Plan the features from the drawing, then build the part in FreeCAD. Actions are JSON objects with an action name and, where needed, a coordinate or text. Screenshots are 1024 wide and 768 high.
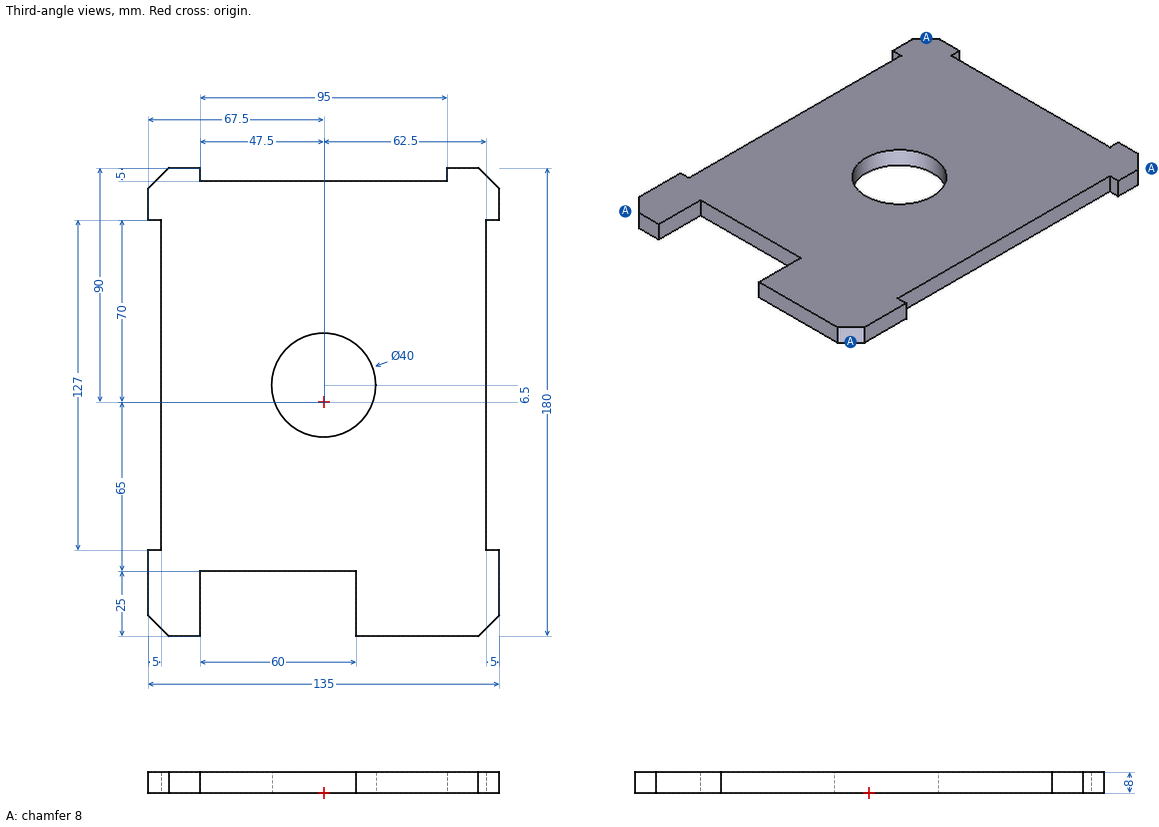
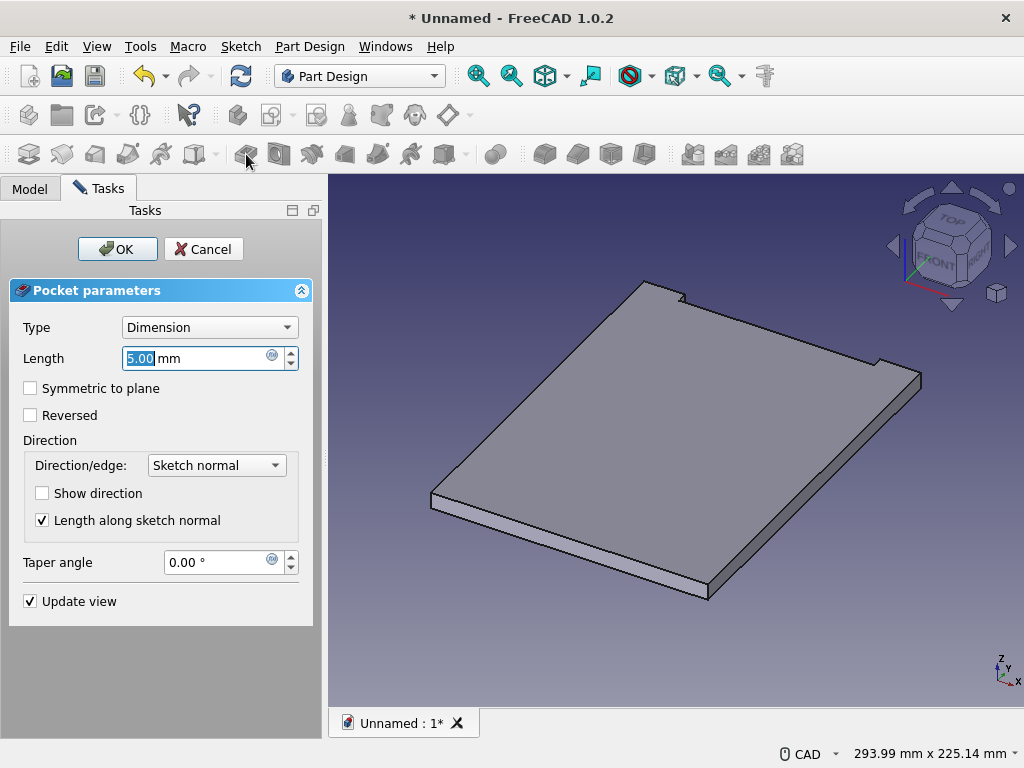
{"action": "left_click", "coordinate": [210, 328]}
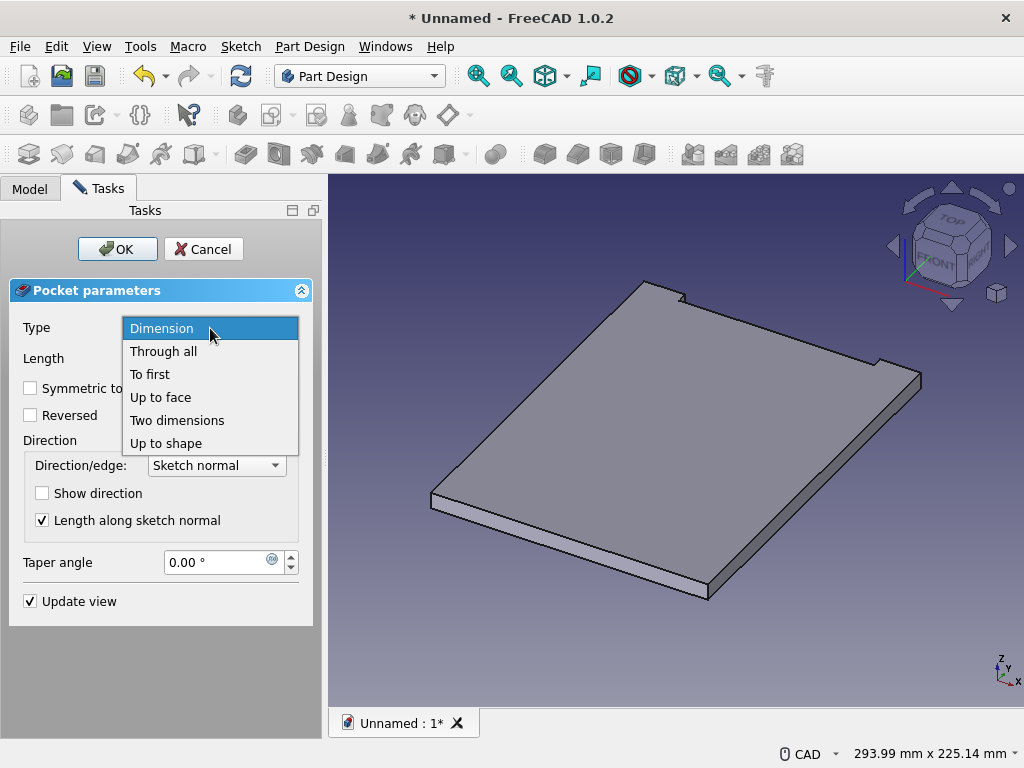
{"action": "left_click", "coordinate": [208, 374]}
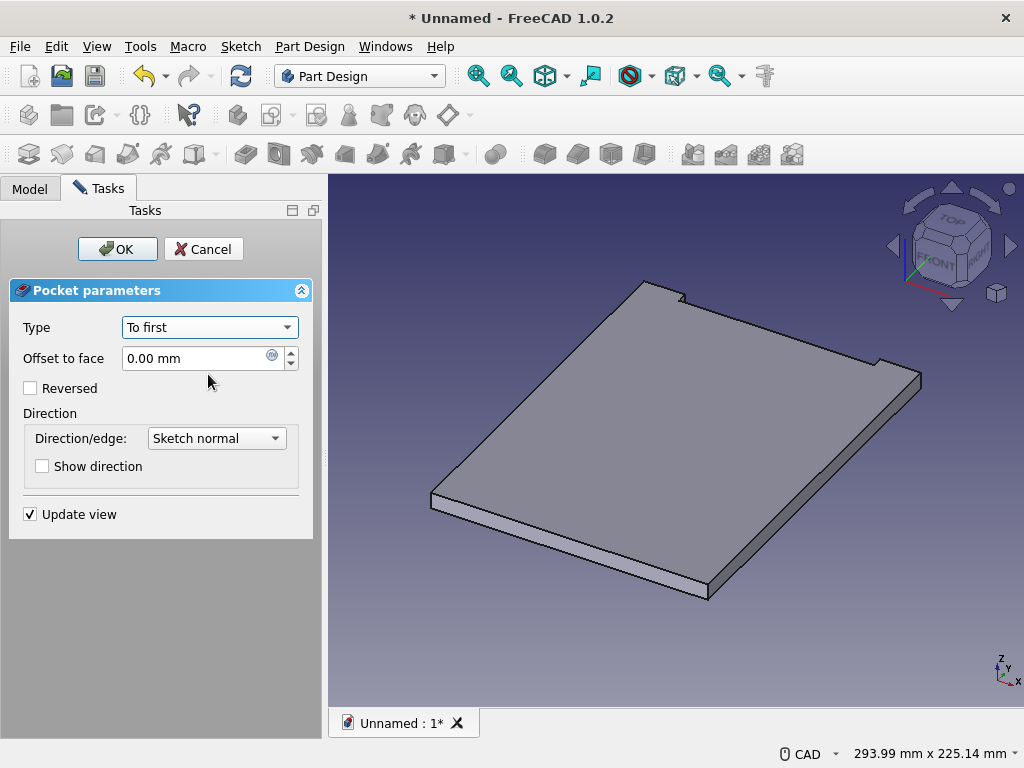
{"action": "left_click", "coordinate": [118, 249]}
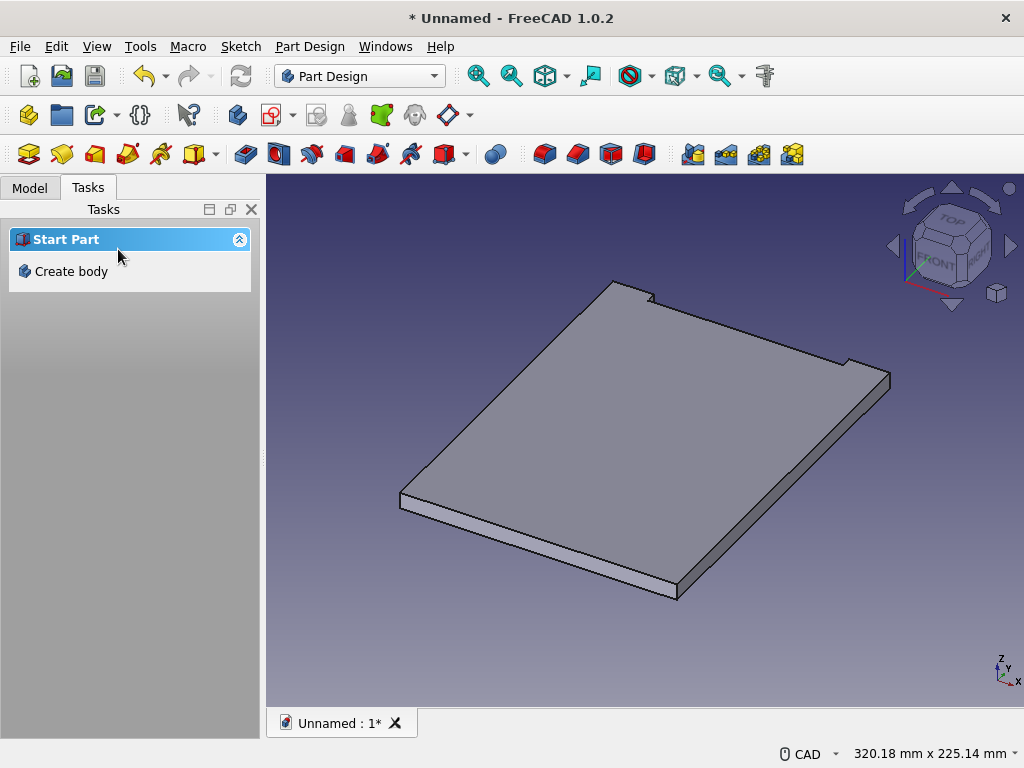
{"action": "left_click", "coordinate": [645, 432]}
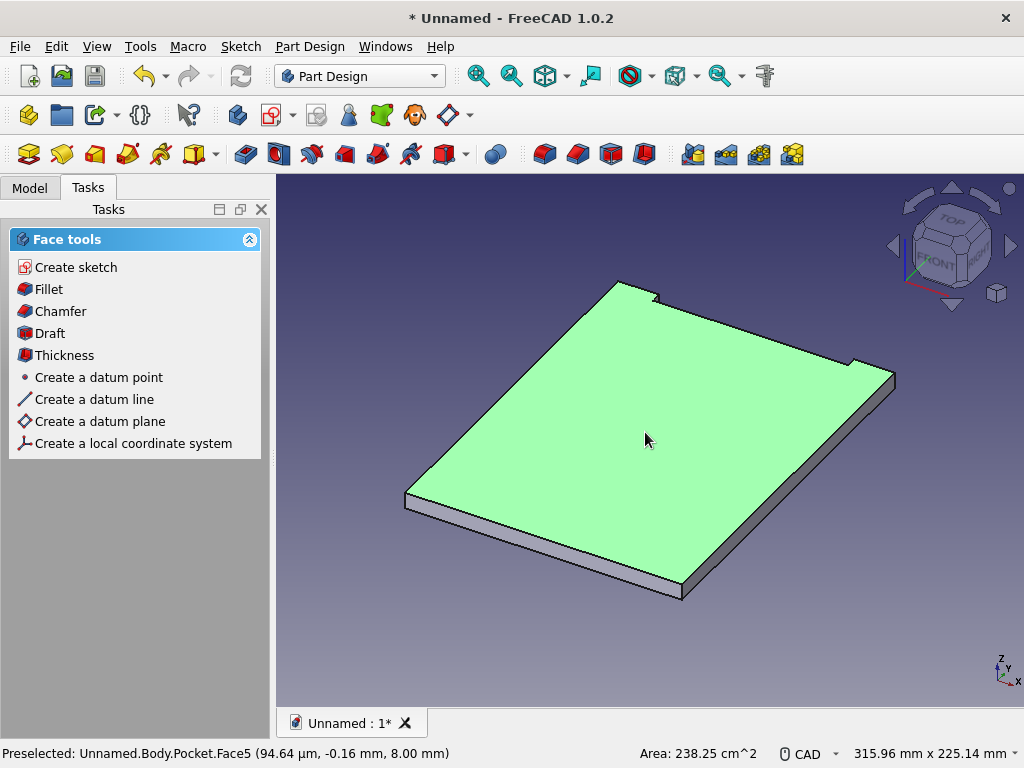
{"action": "left_click", "coordinate": [270, 116]}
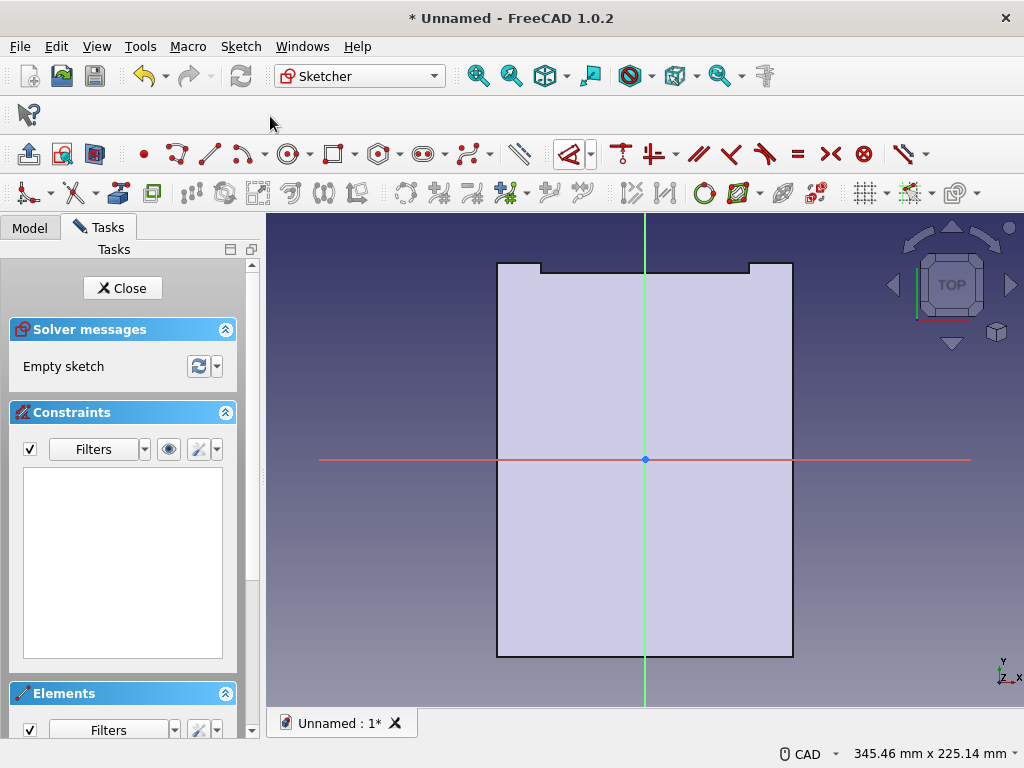
{"action": "scroll", "coordinate": [668, 679], "scroll_direction": "up", "scroll_amount": 2}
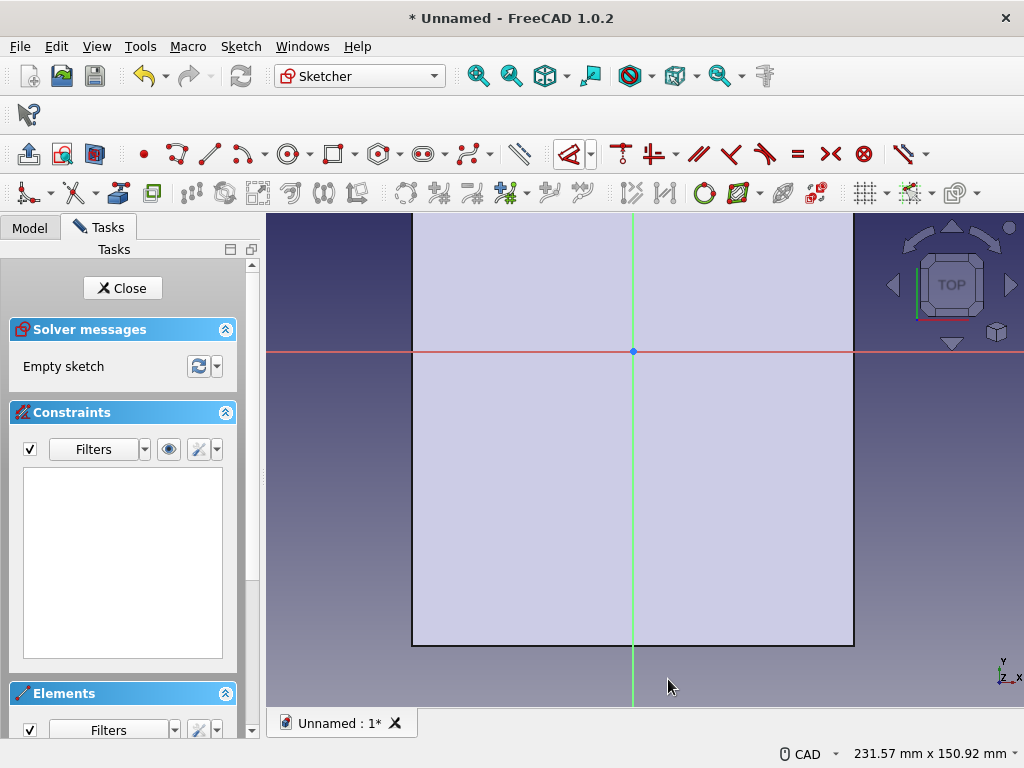
{"action": "left_click", "coordinate": [332, 154]}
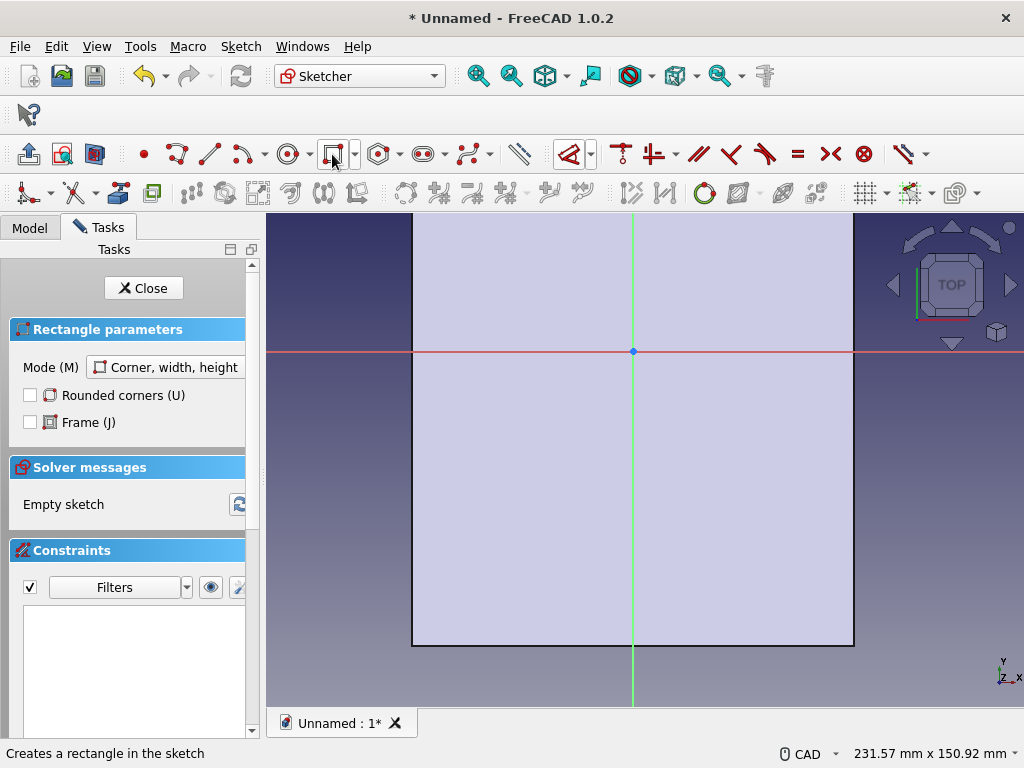
{"action": "left_click", "coordinate": [478, 565]}
{"action": "left_click", "coordinate": [674, 646]}
{"action": "key", "text": "Escape"}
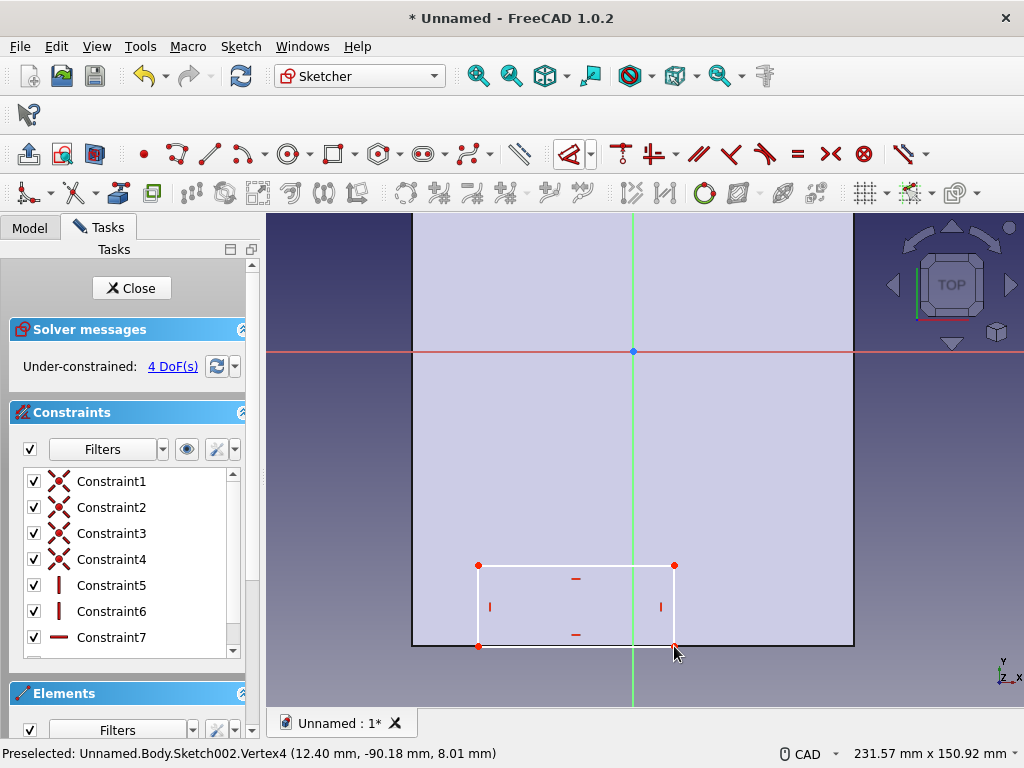
{"action": "left_click", "coordinate": [478, 590]}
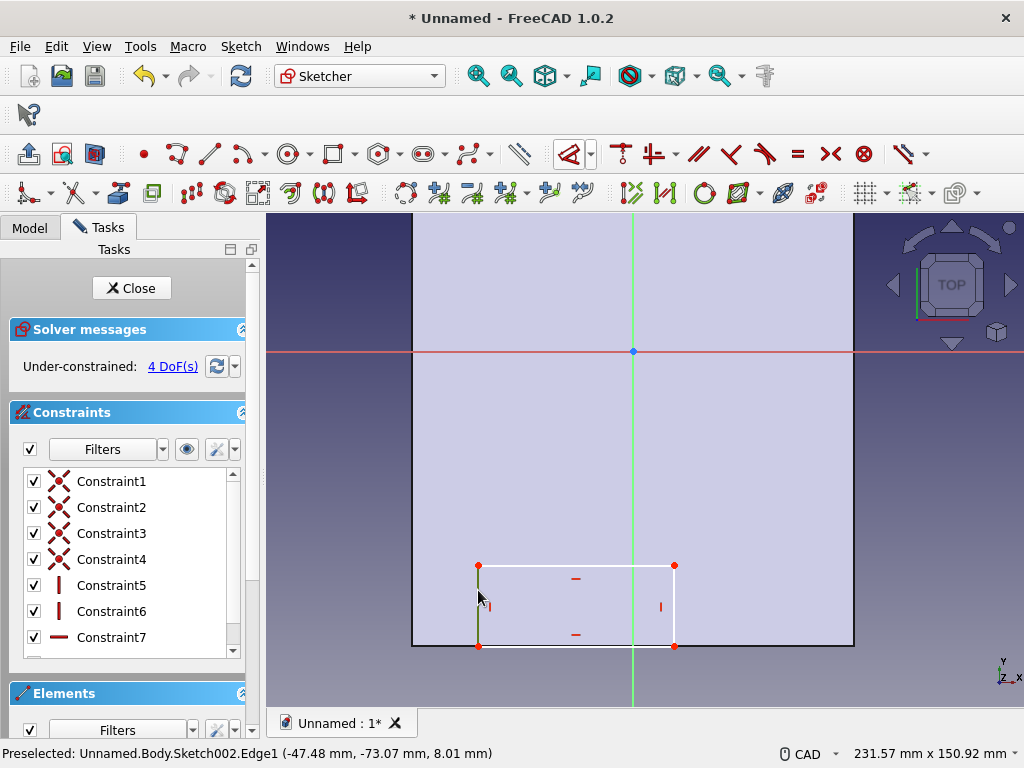
{"action": "key", "text": "i"}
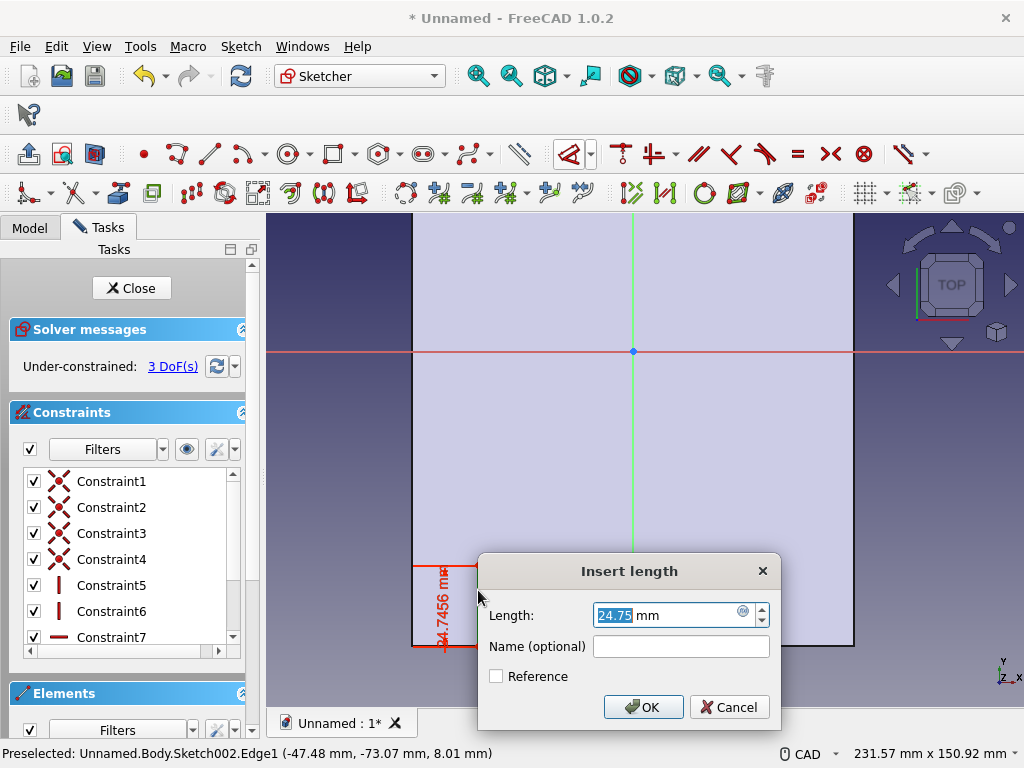
{"action": "type", "text": "25"}
{"action": "key", "text": "Return"}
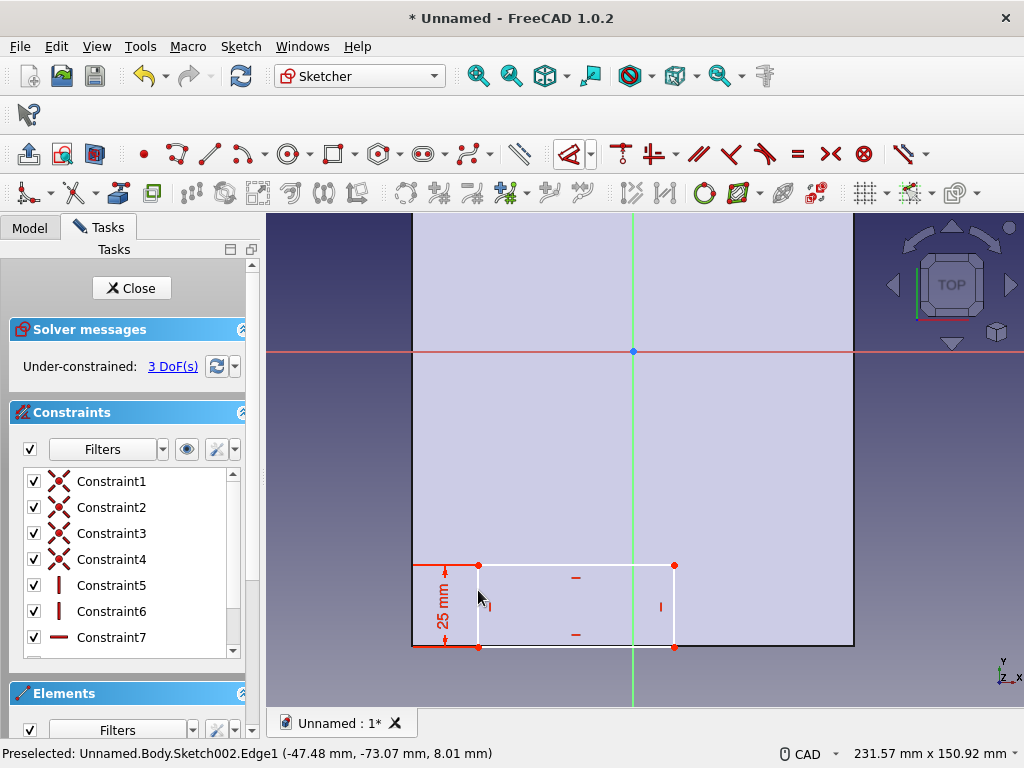
{"action": "left_click", "coordinate": [537, 647]}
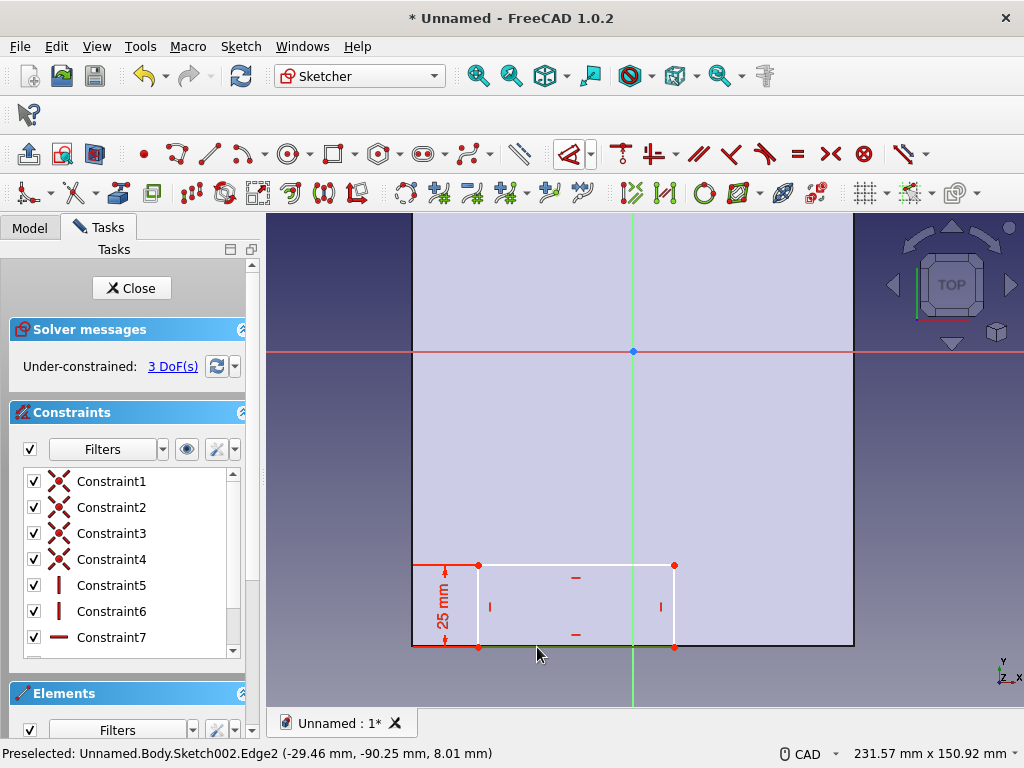
{"action": "key", "text": "l"}